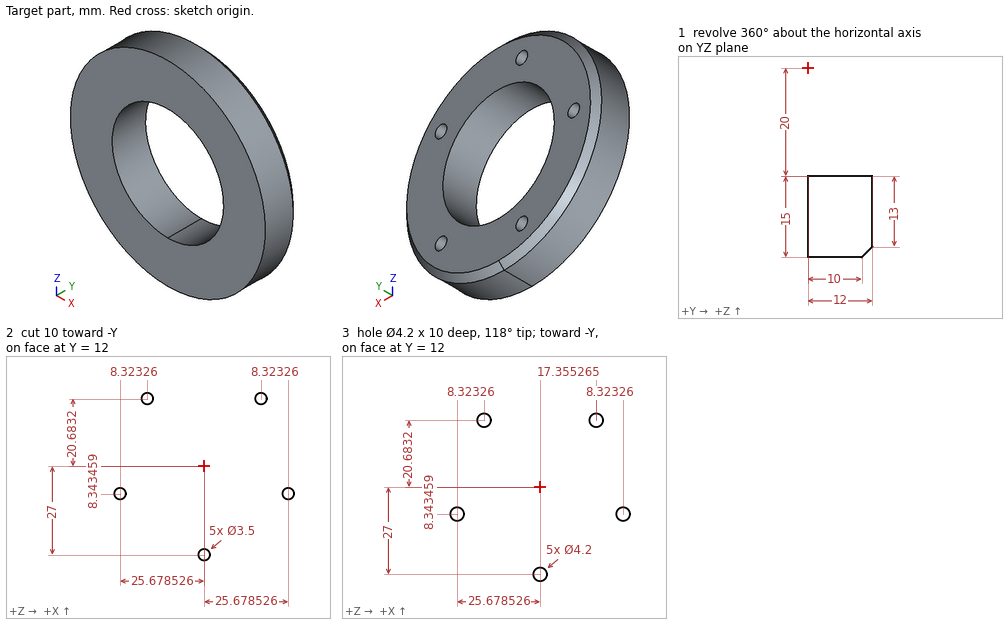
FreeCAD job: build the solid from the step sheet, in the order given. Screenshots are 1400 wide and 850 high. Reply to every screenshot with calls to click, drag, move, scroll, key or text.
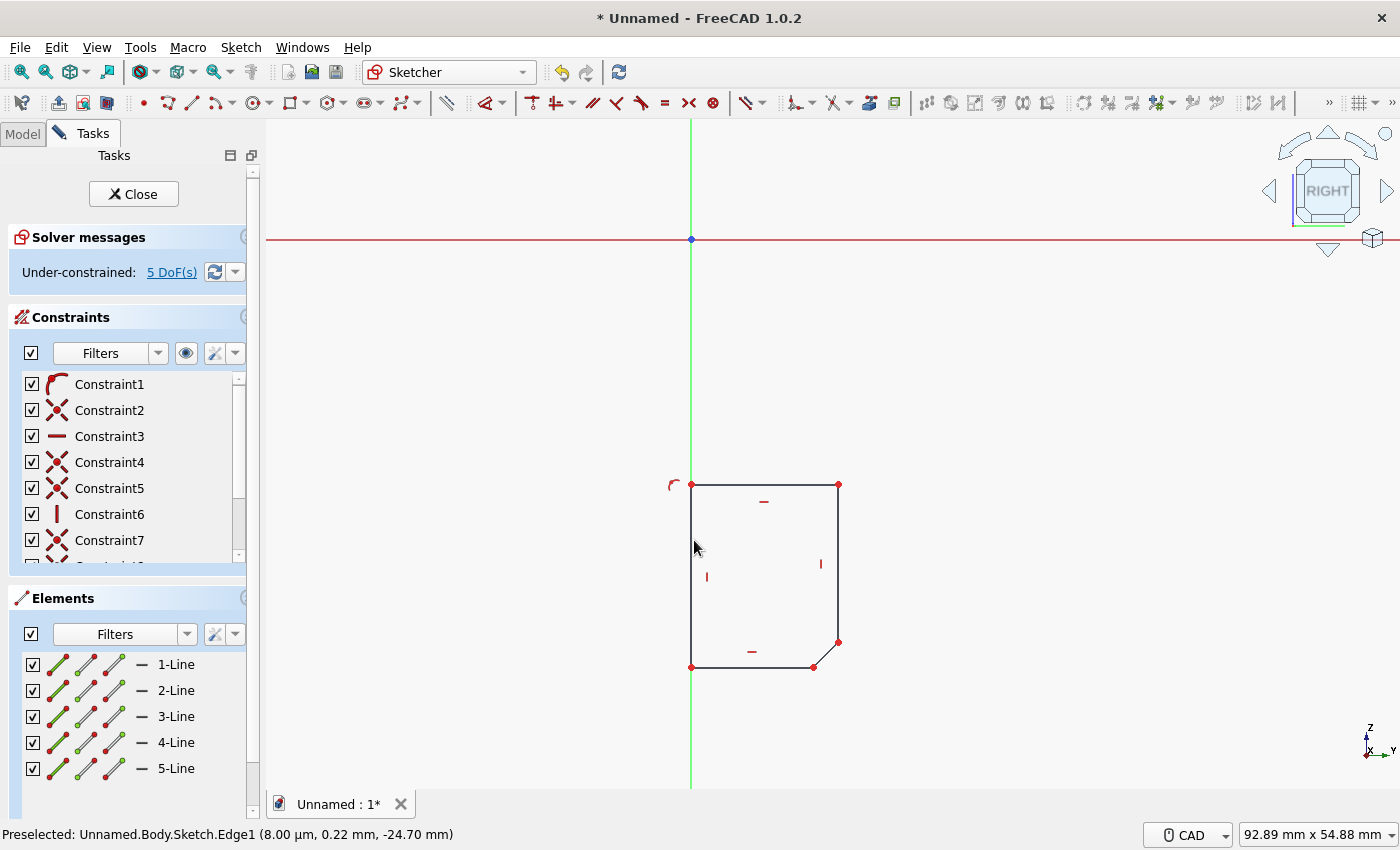
key(d)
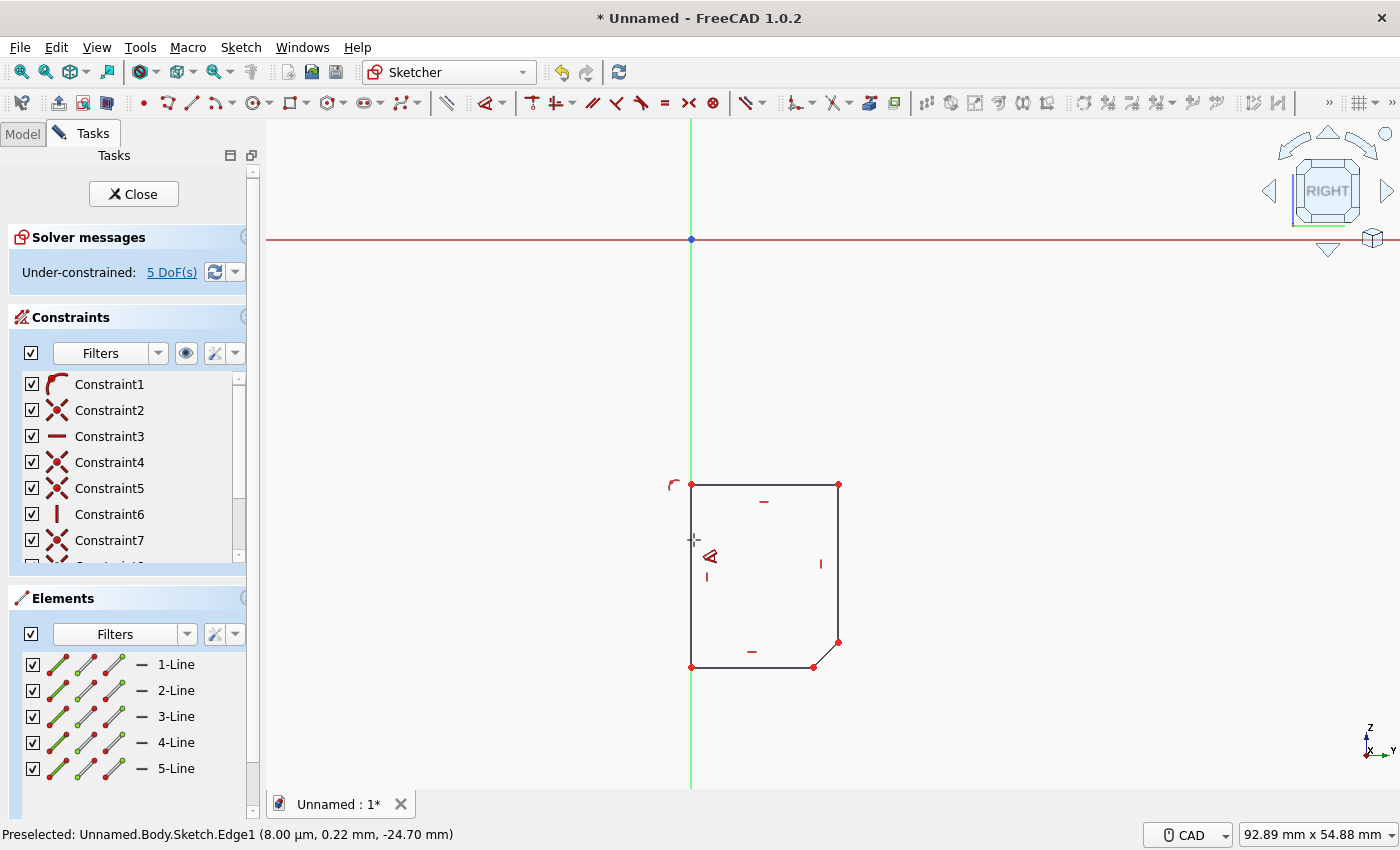
click(691, 540)
click(657, 576)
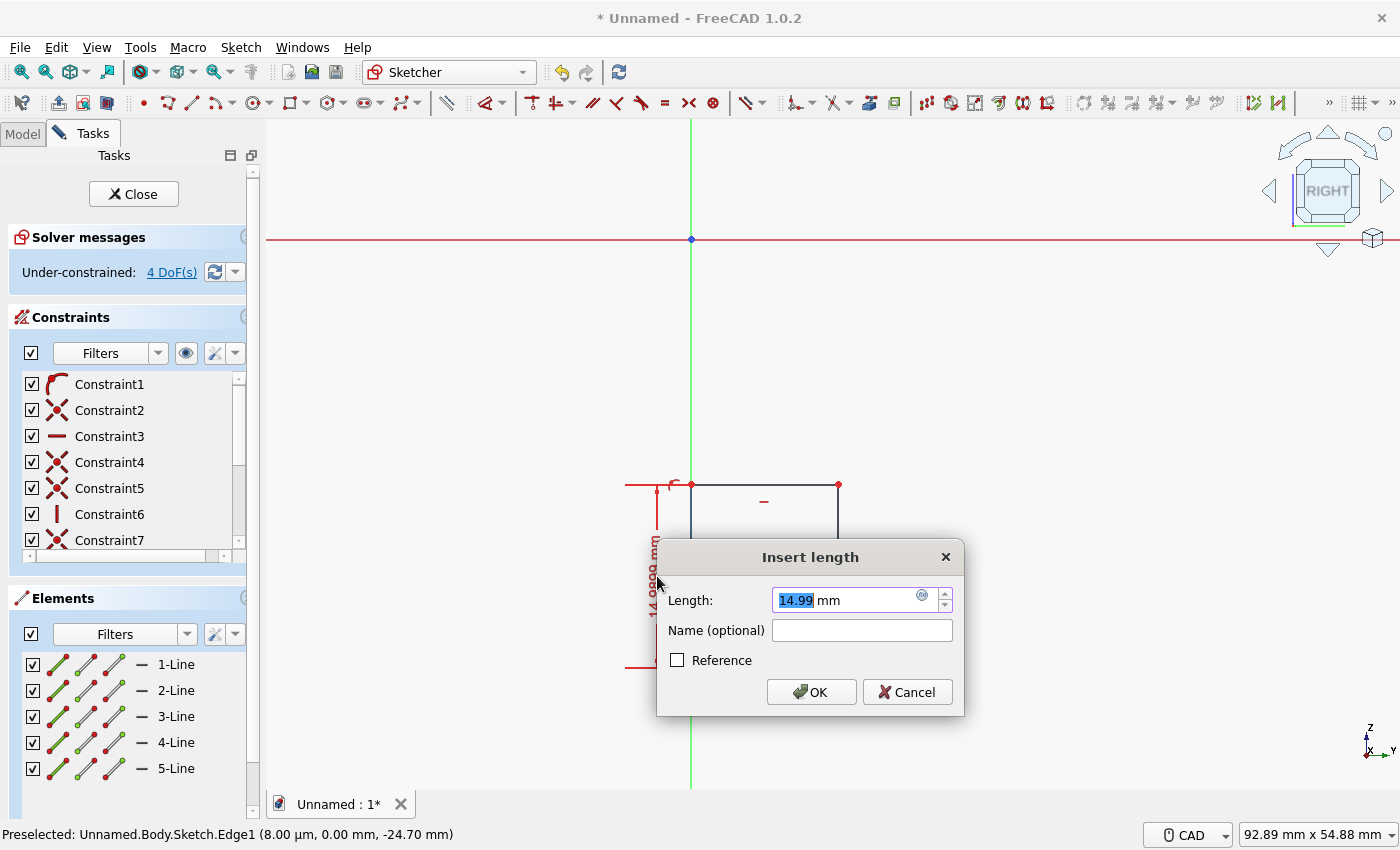
text(15)
key(Return)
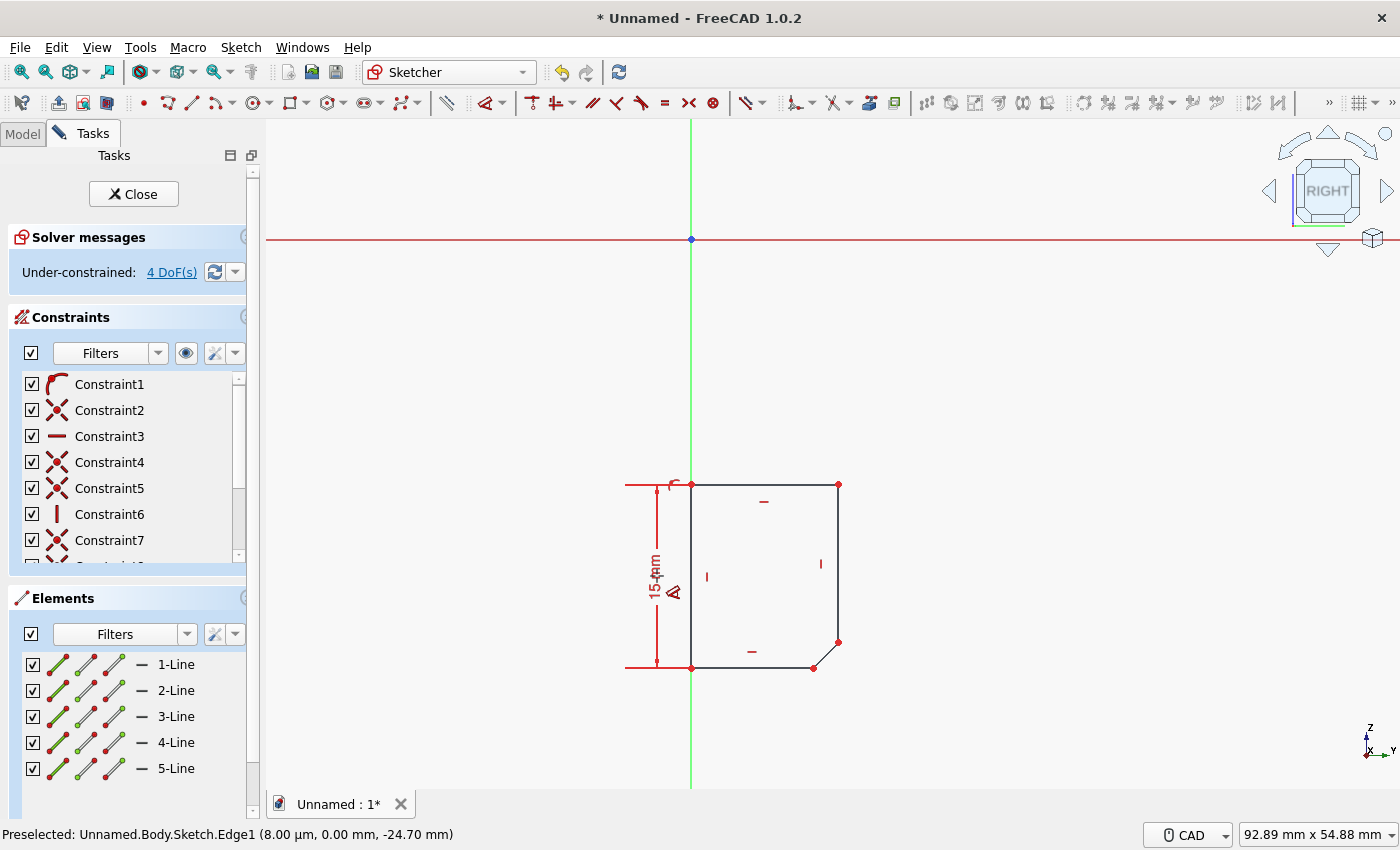
click(728, 668)
click(752, 702)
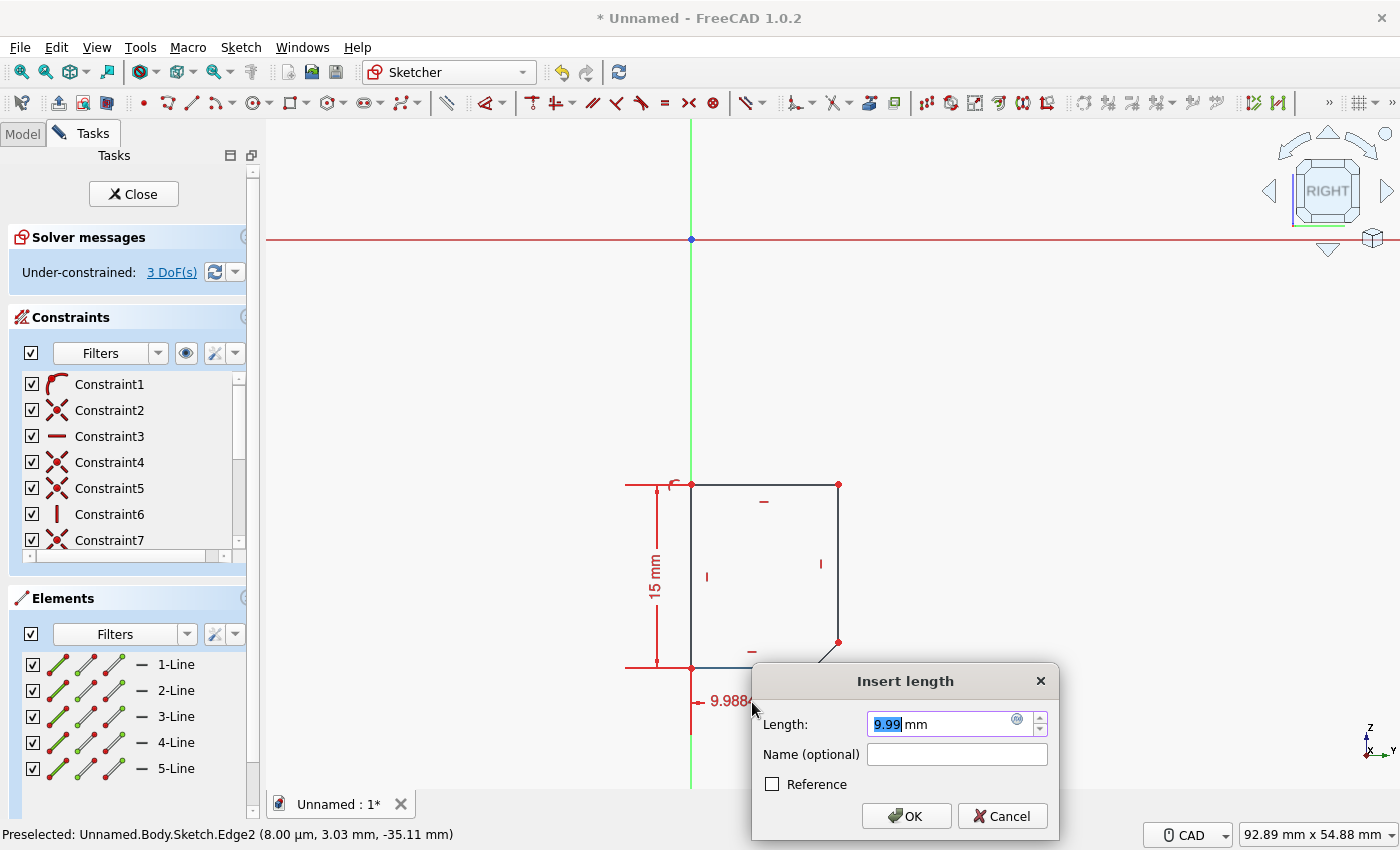
text(10)
key(Return)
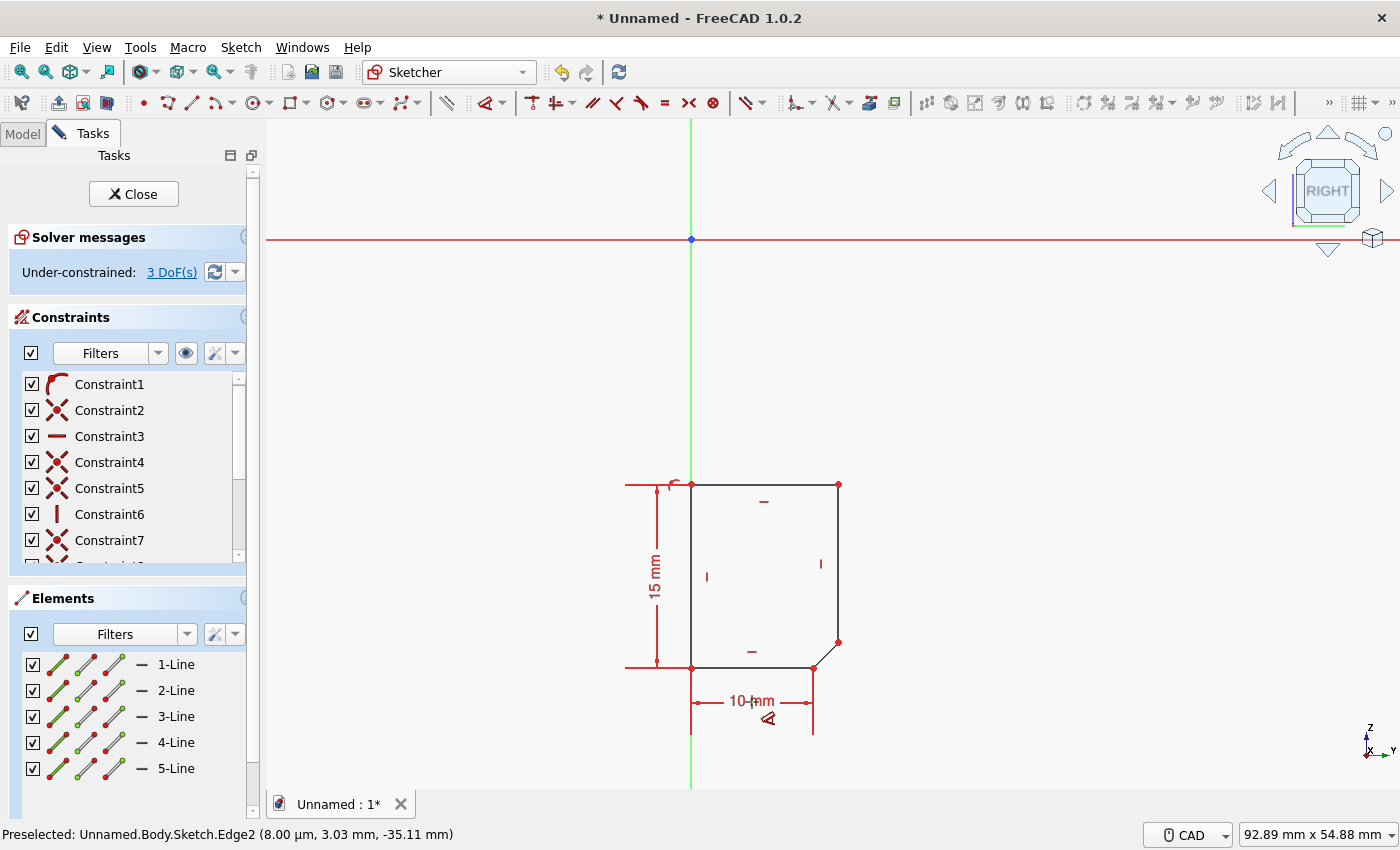
click(838, 596)
click(872, 564)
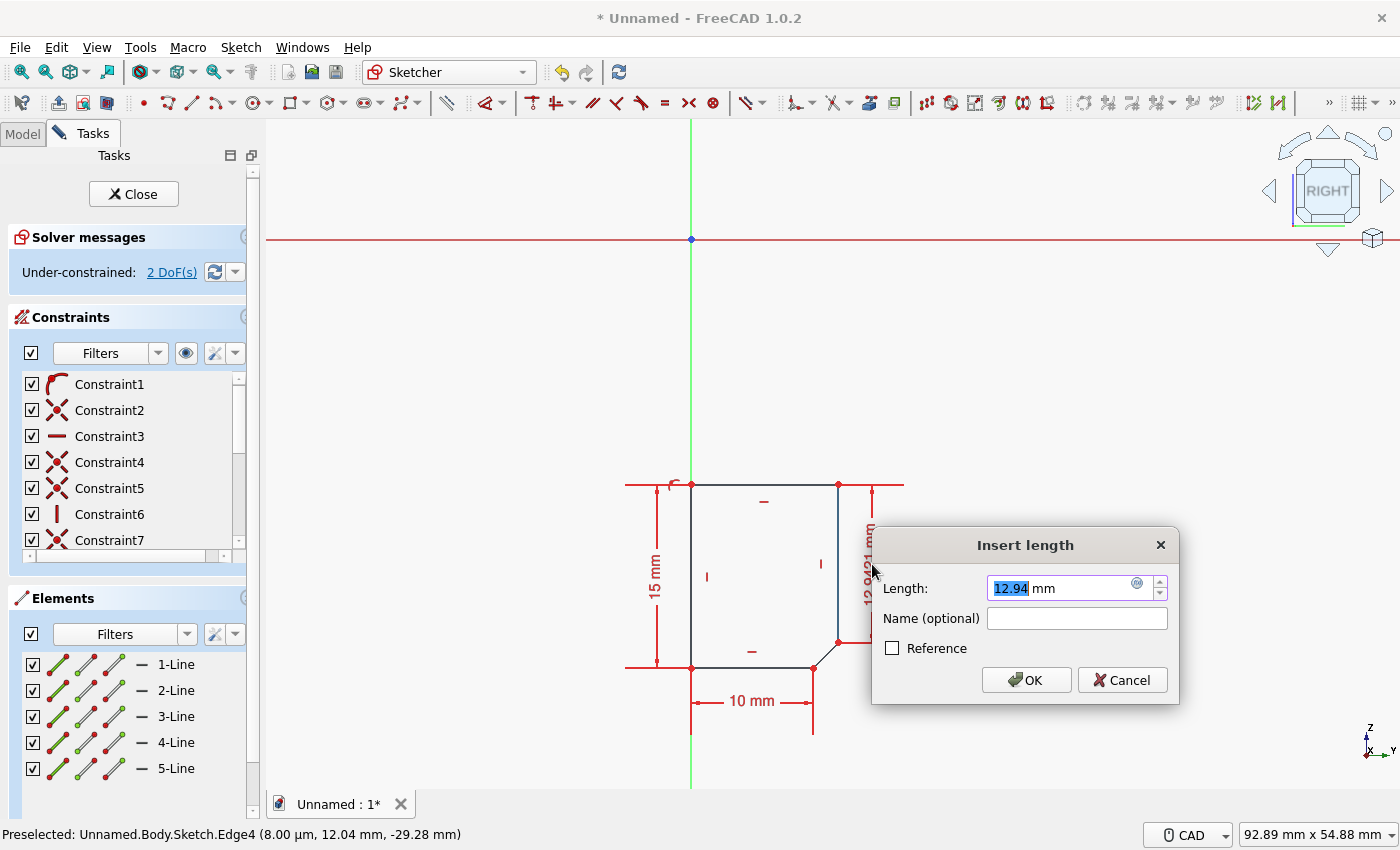
text(13)
key(Return)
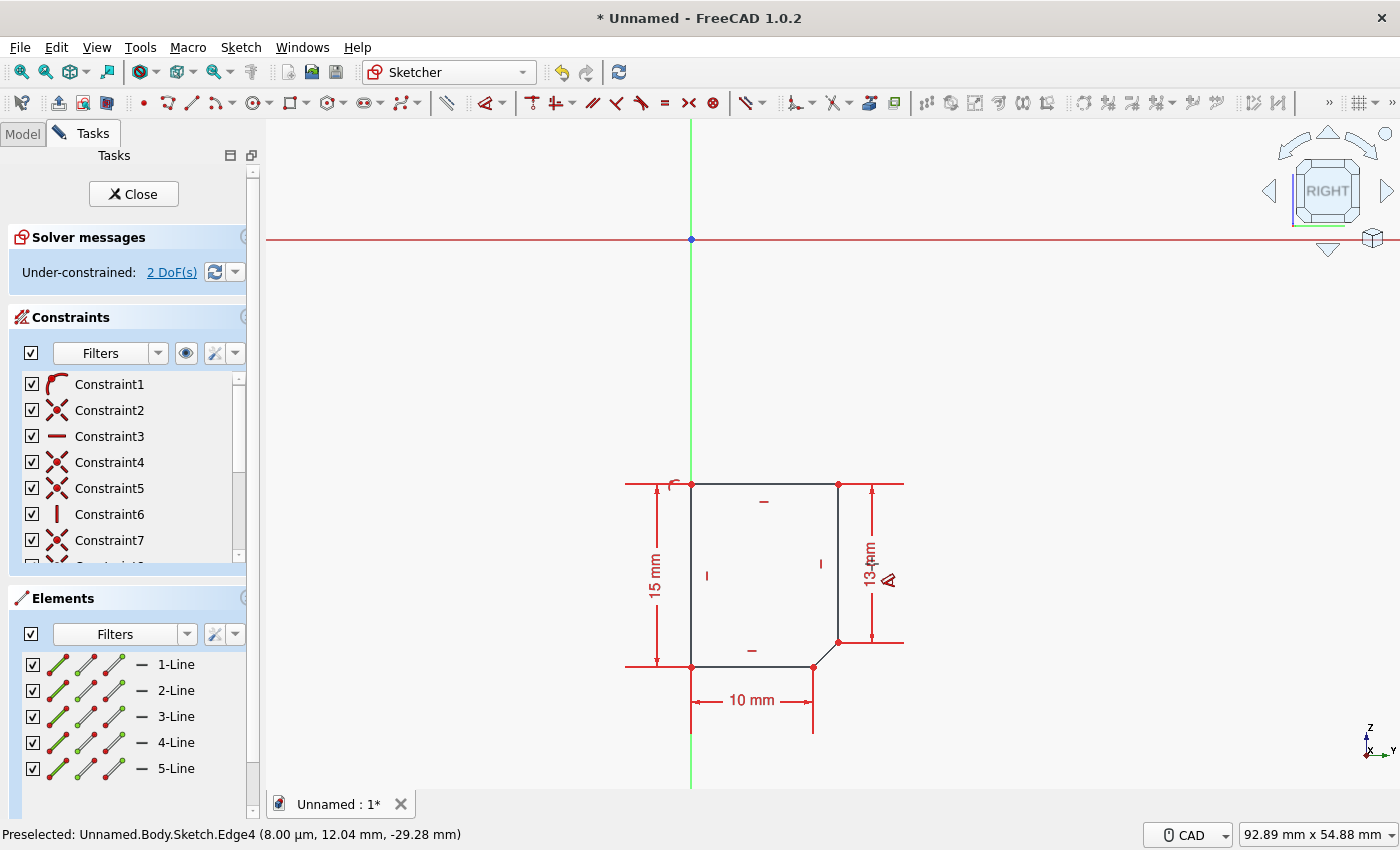
click(794, 484)
click(765, 518)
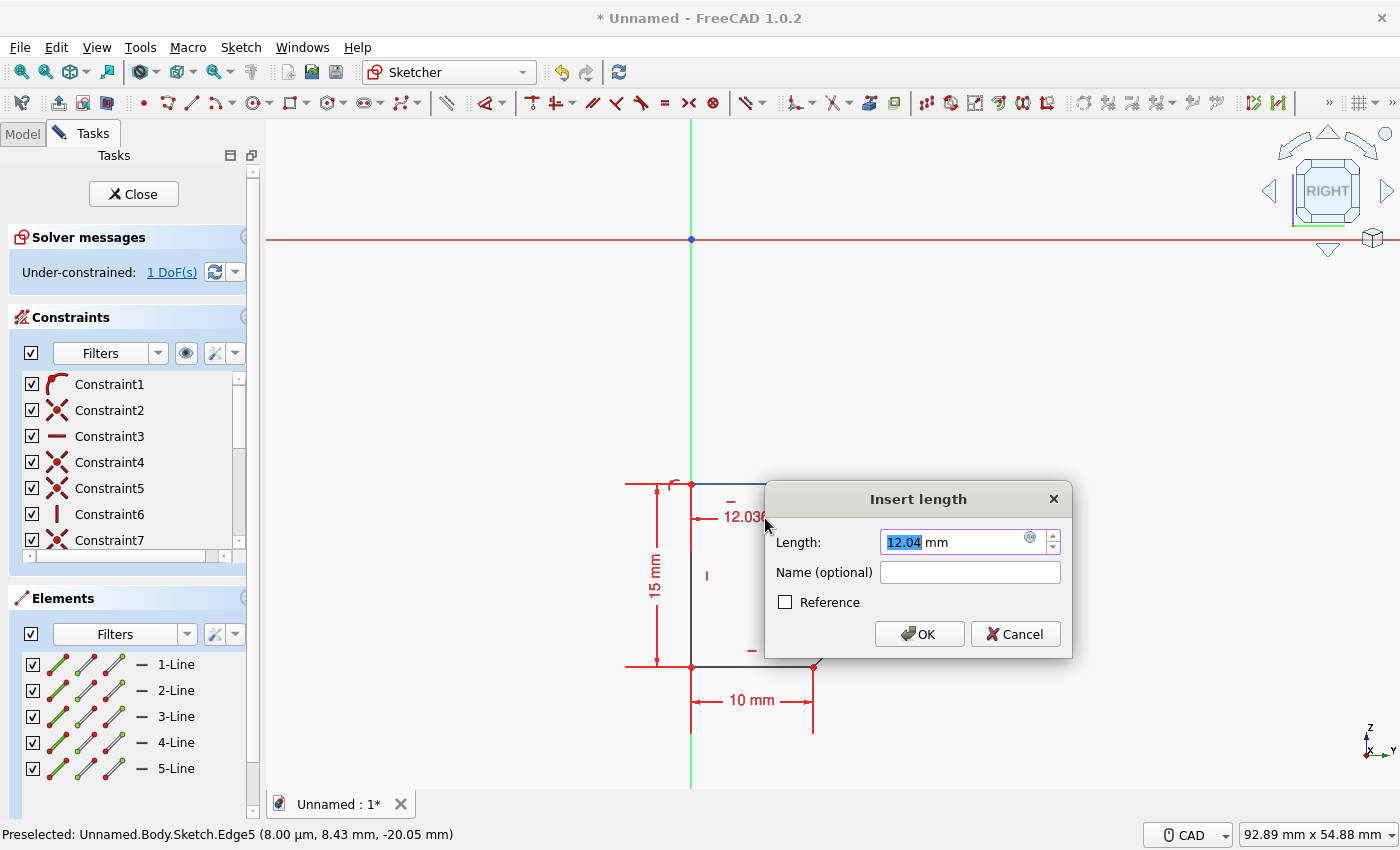
text(12)
key(Return)